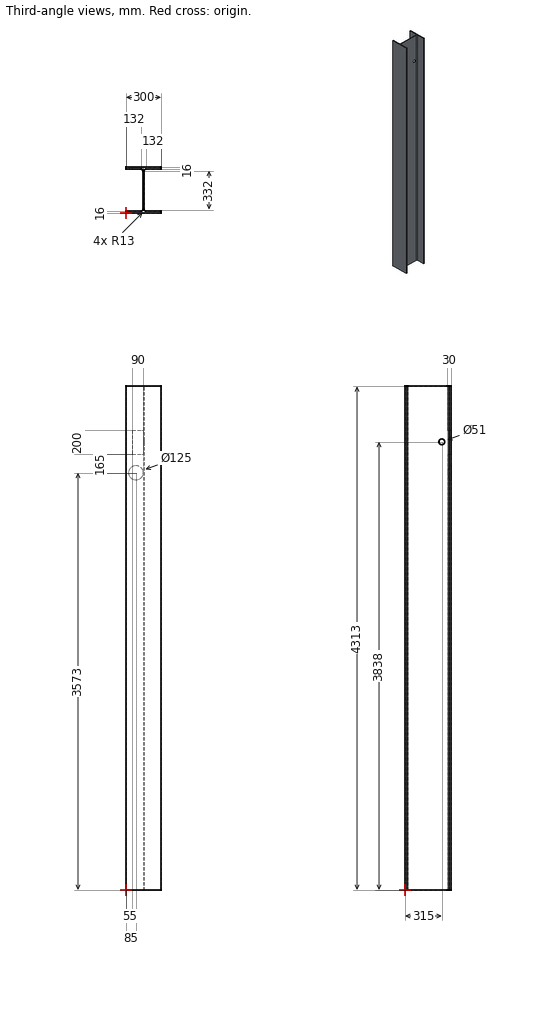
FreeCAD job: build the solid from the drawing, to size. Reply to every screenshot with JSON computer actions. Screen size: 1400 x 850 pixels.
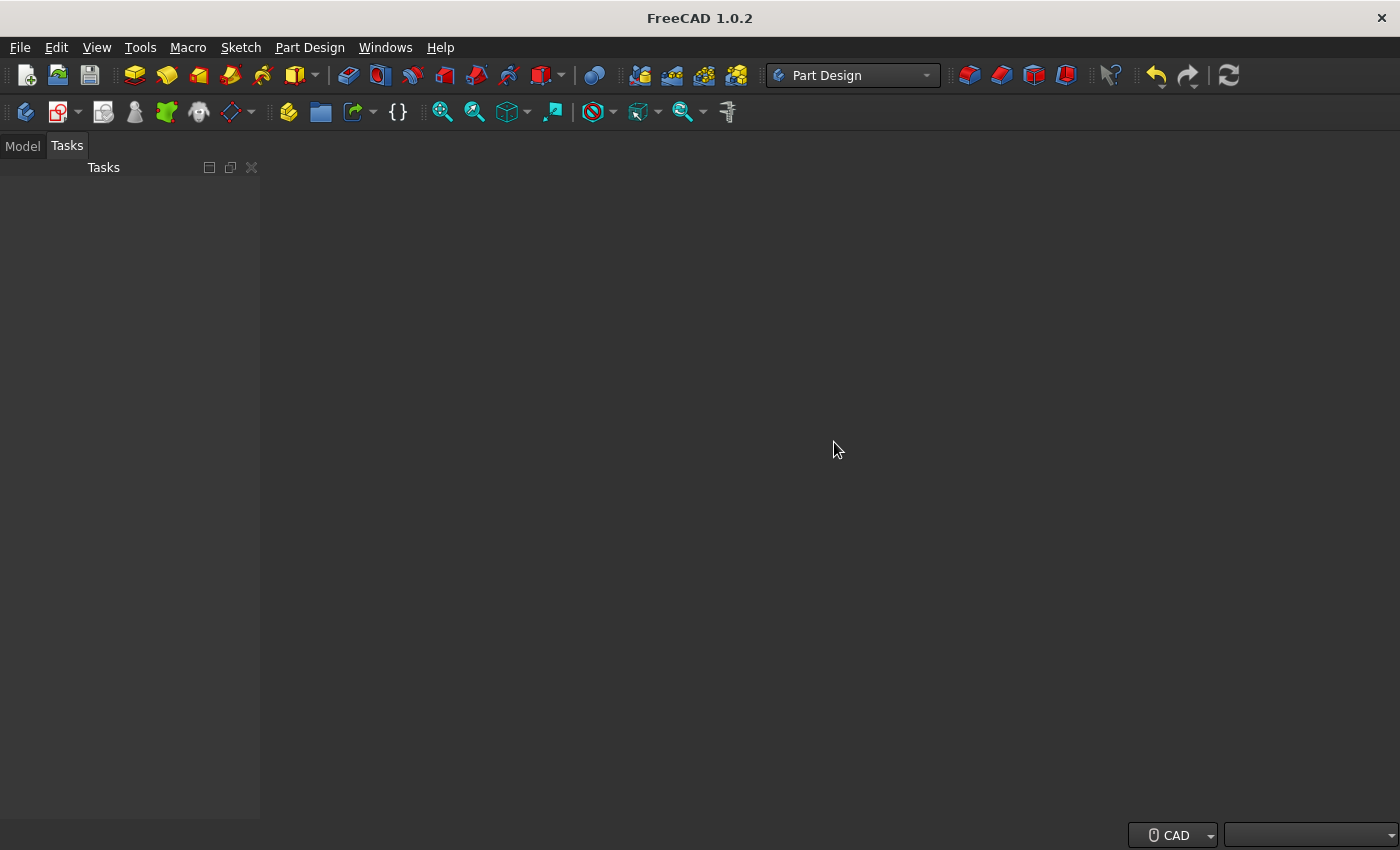
{"action": "left_click", "coordinate": [26, 76]}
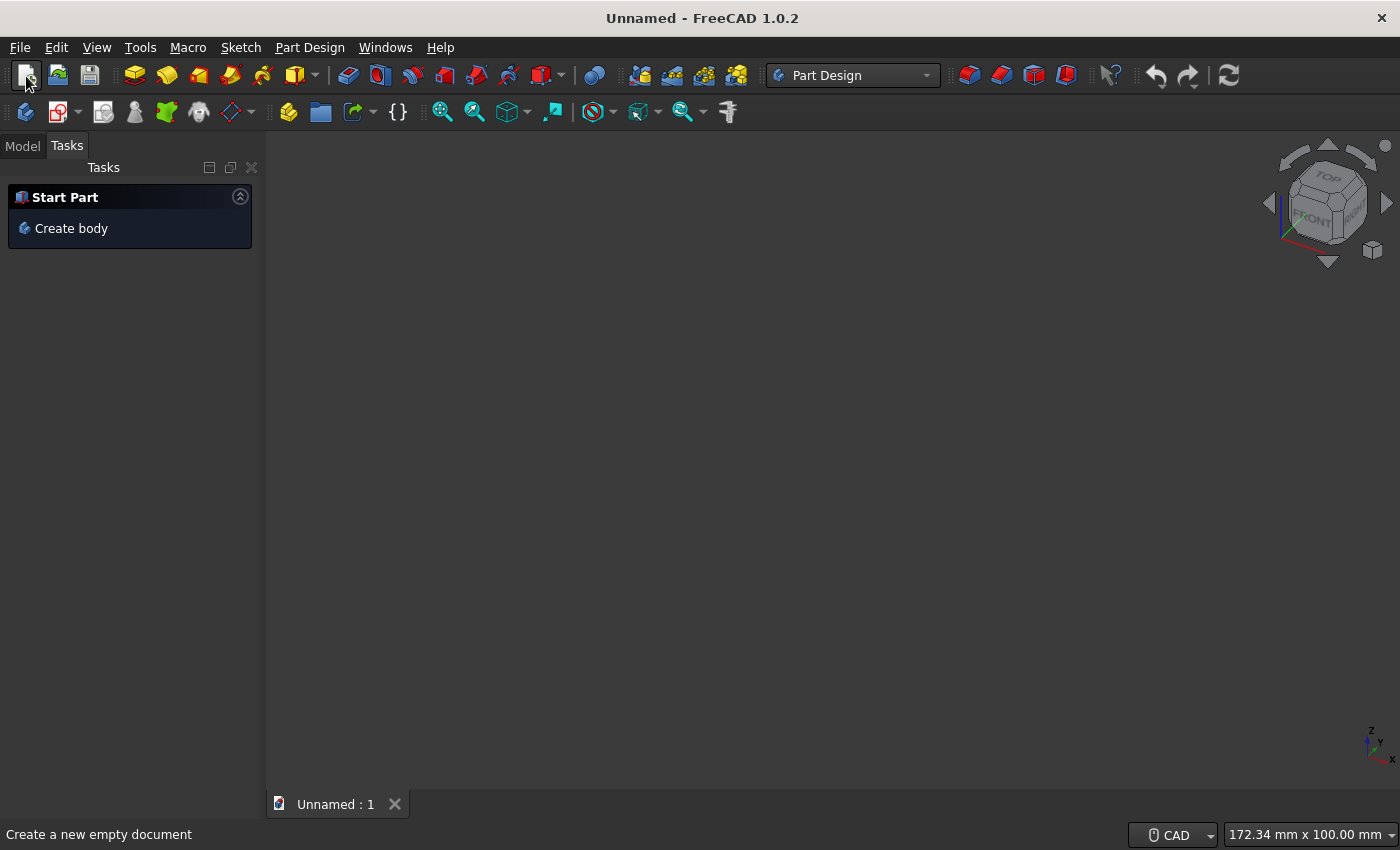
{"action": "left_click", "coordinate": [58, 112]}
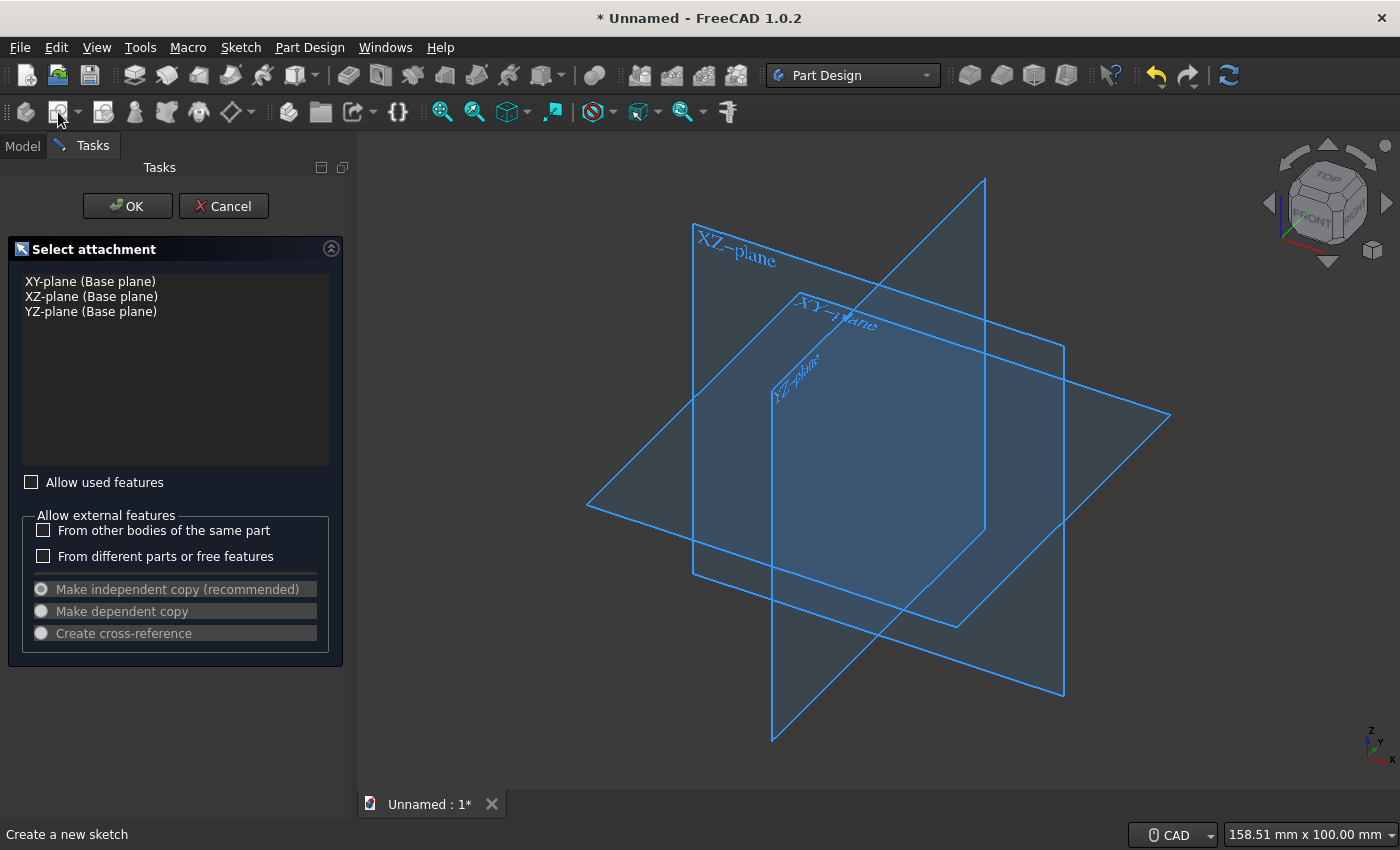
{"action": "left_click", "coordinate": [82, 282]}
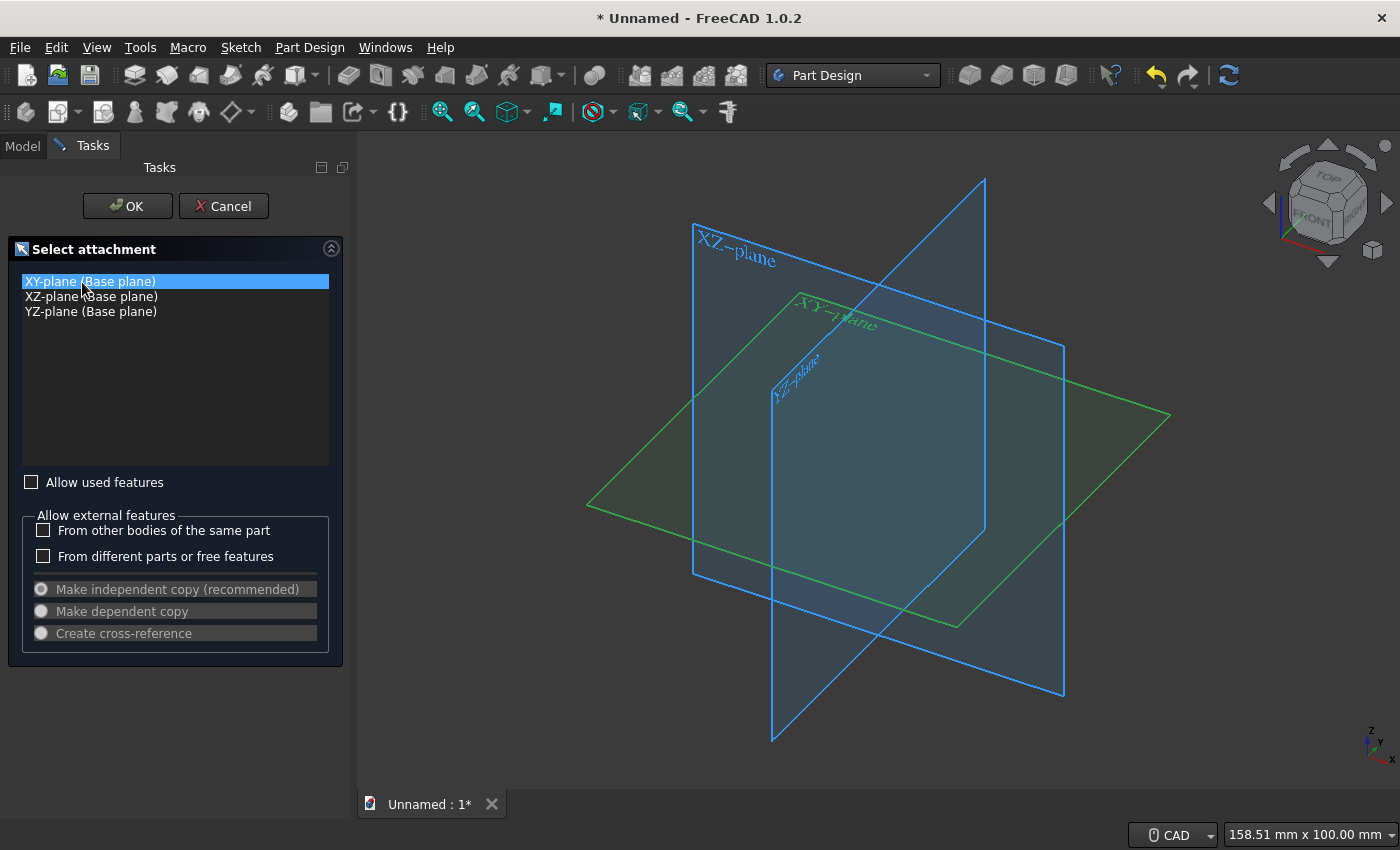
{"action": "left_click", "coordinate": [128, 206]}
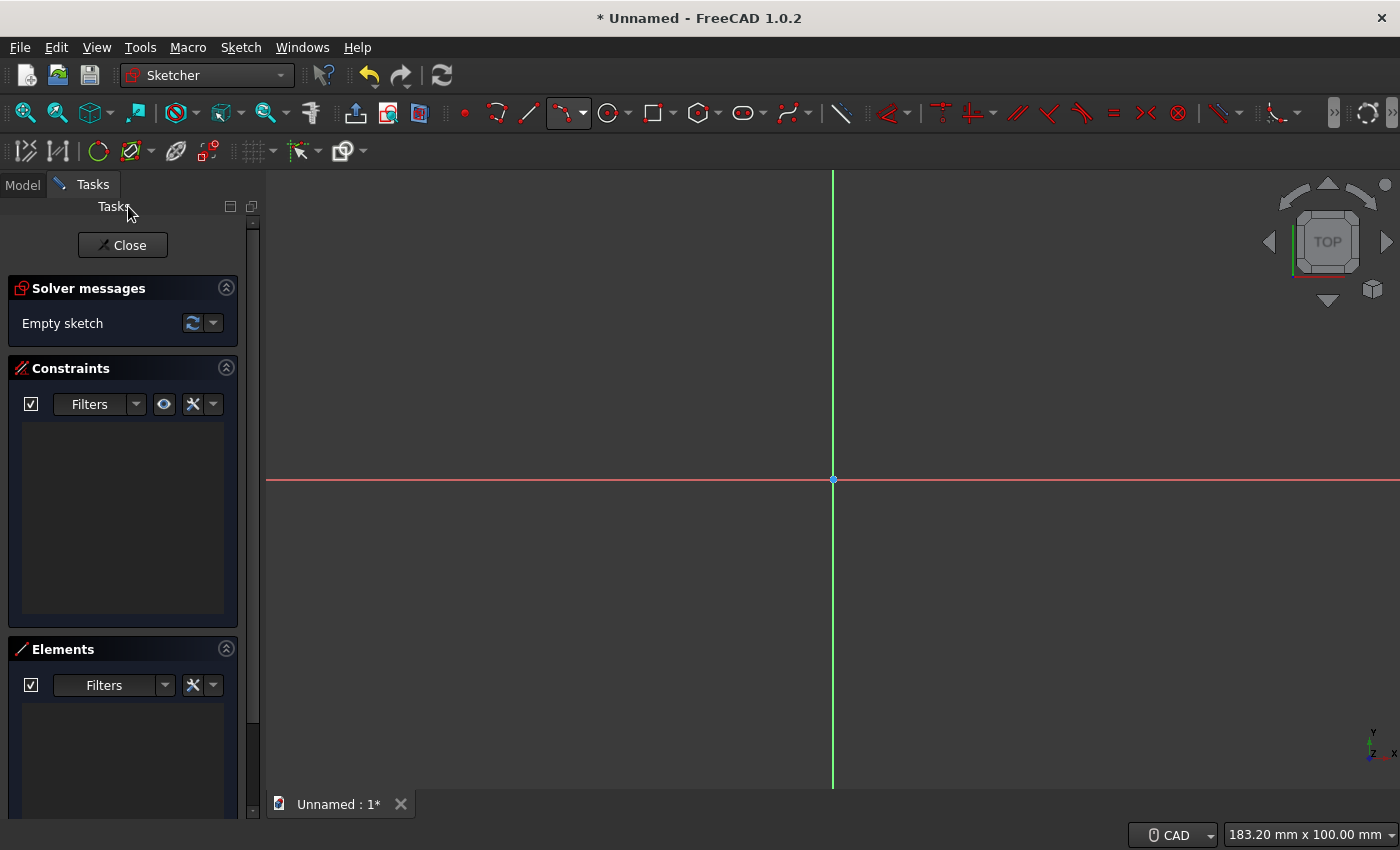
{"action": "scroll", "coordinate": [567, 719], "scroll_direction": "down", "scroll_amount": 9}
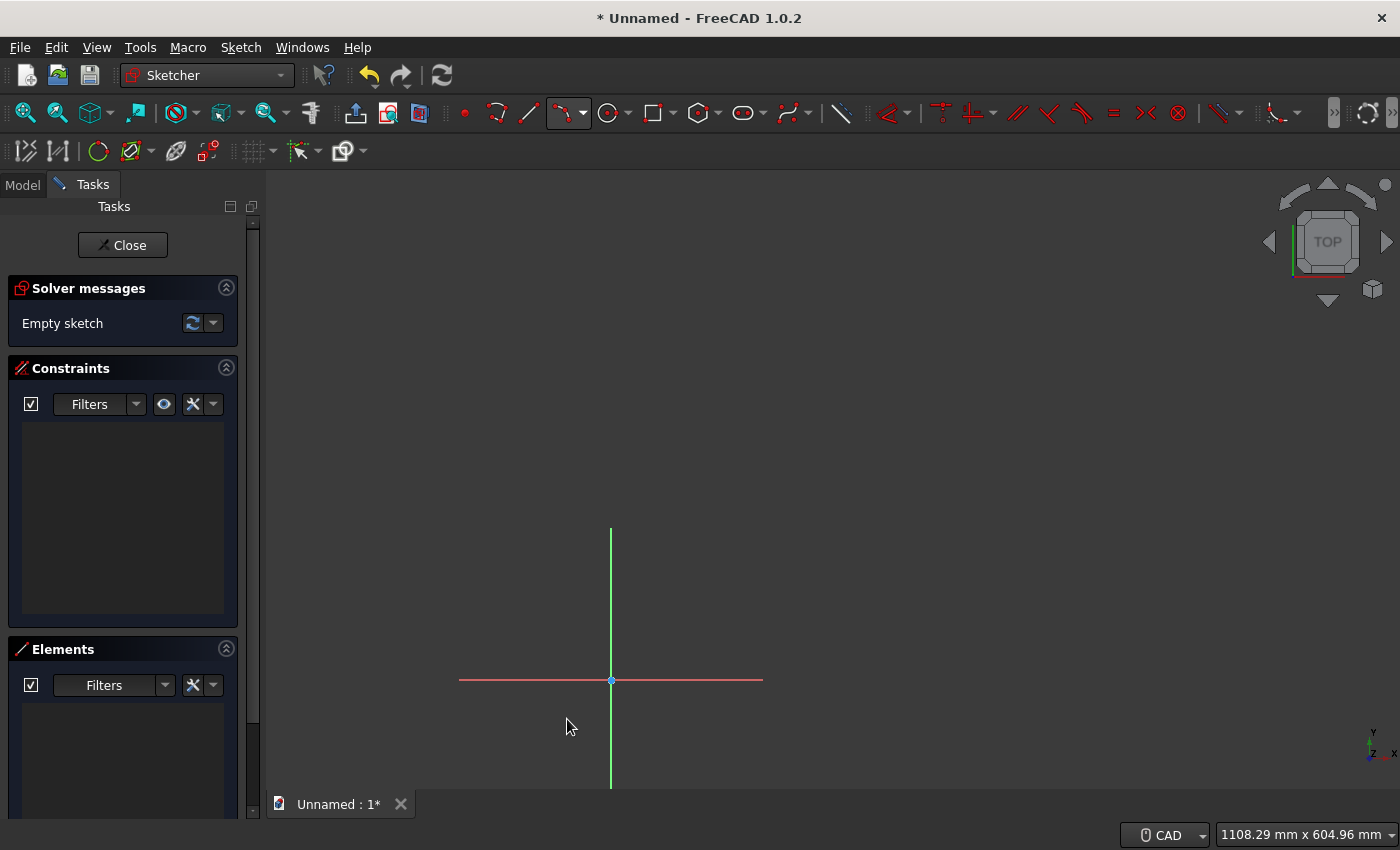
{"action": "key", "text": "g l"}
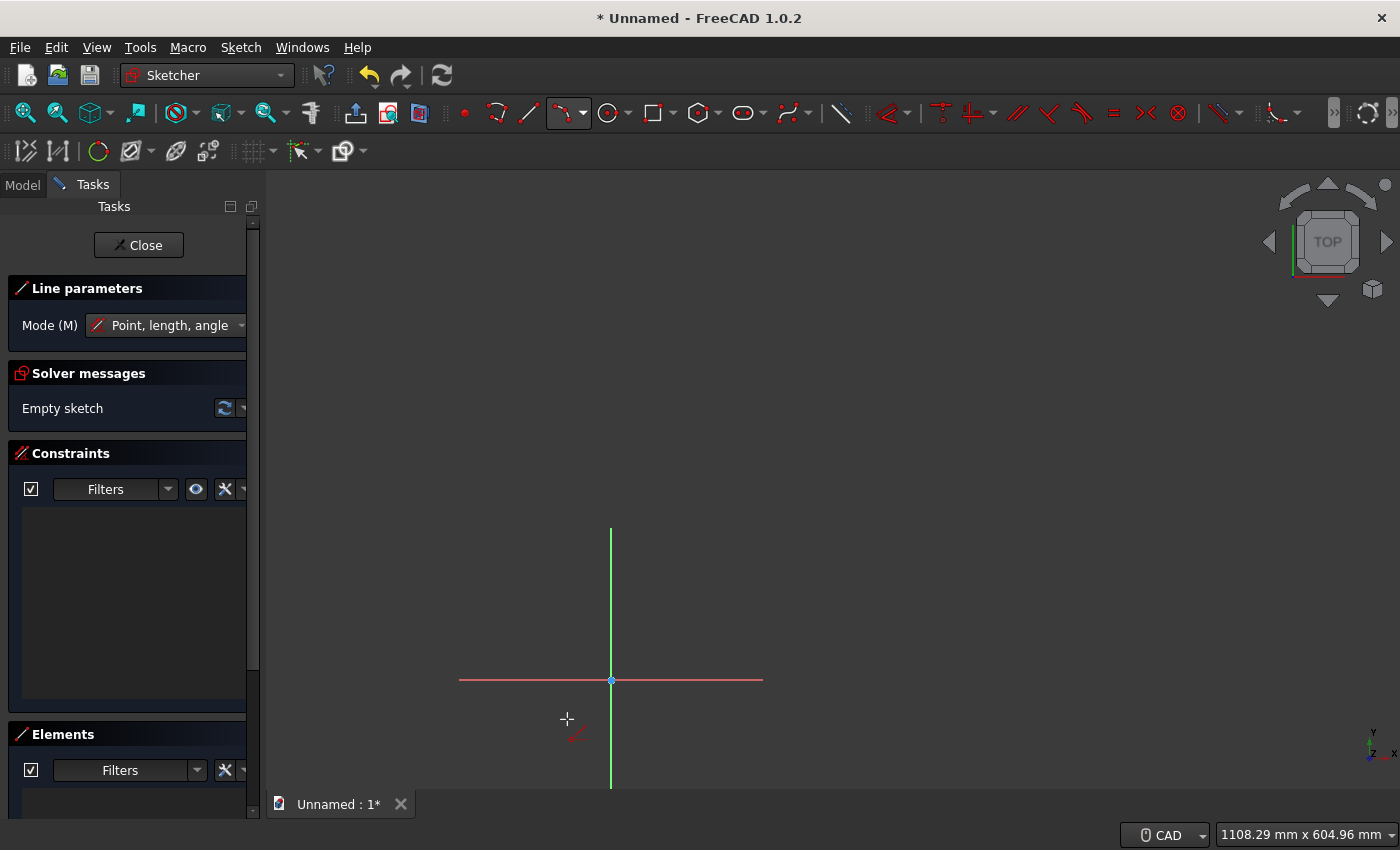
{"action": "left_click", "coordinate": [770, 650]}
{"action": "left_click", "coordinate": [770, 311]}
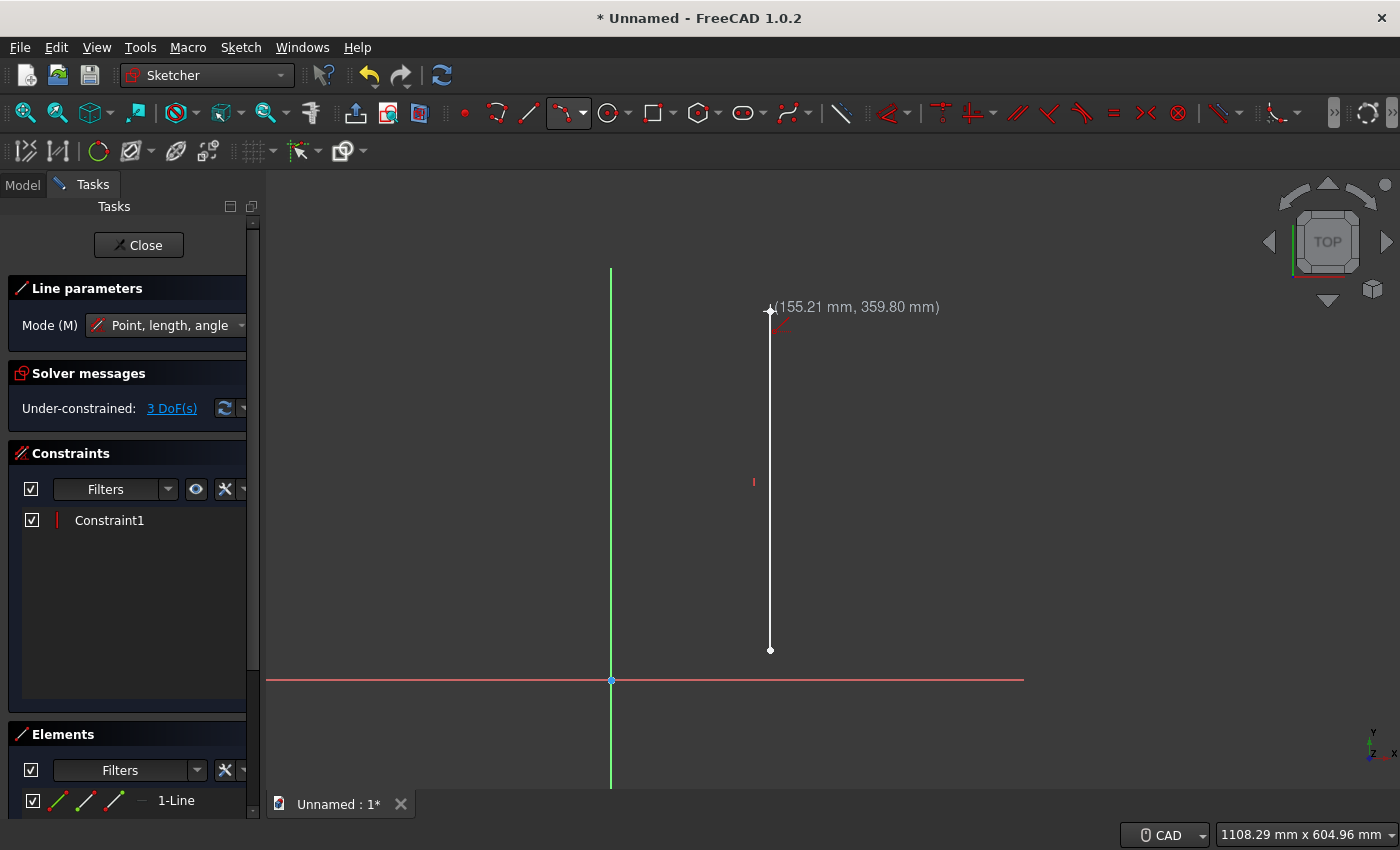
{"action": "left_click", "coordinate": [498, 114]}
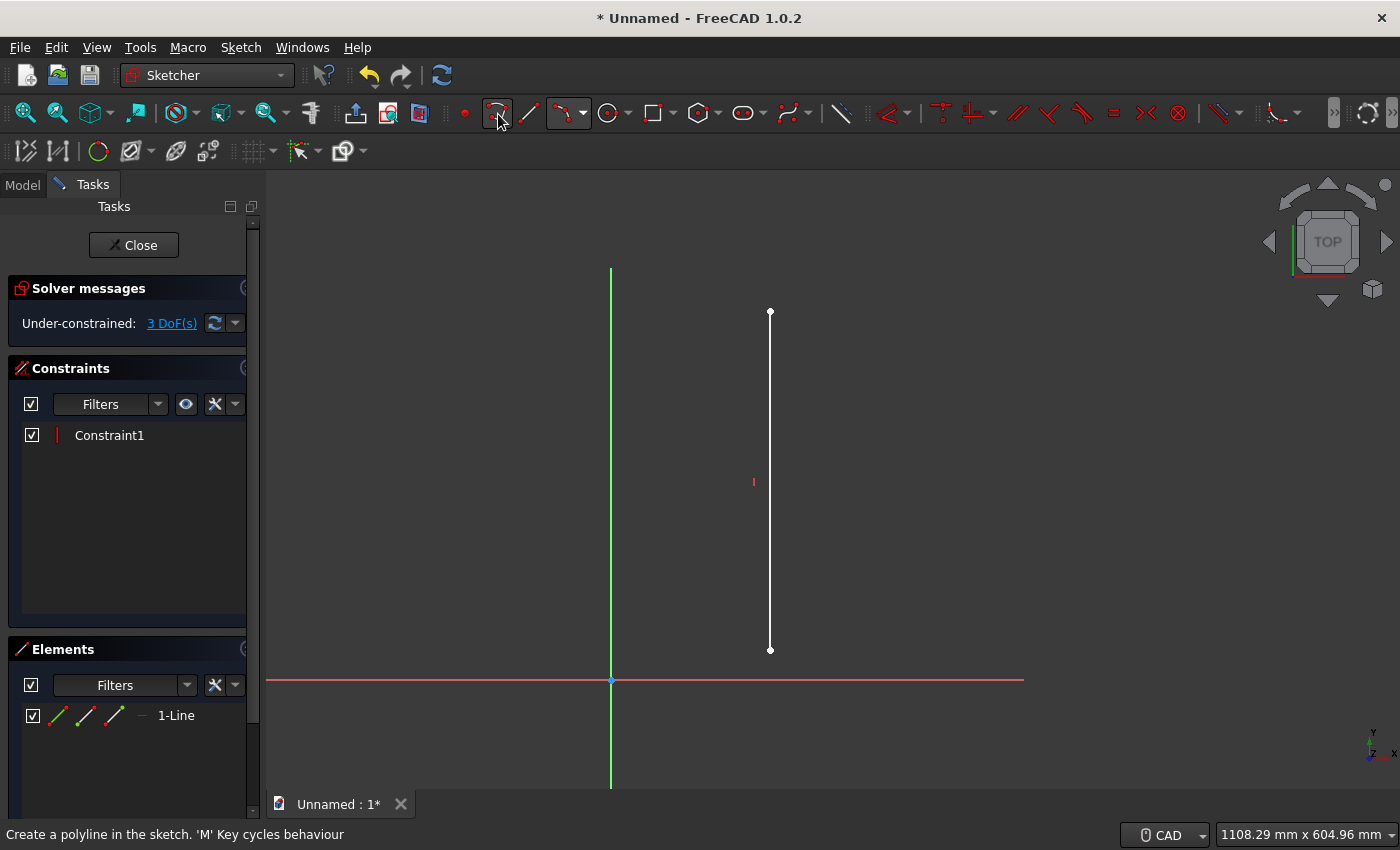
{"action": "left_click", "coordinate": [783, 297]}
{"action": "left_click", "coordinate": [918, 297]}
{"action": "left_click", "coordinate": [918, 281]}
{"action": "left_click", "coordinate": [611, 281]}
{"action": "left_click", "coordinate": [620, 297]}
{"action": "left_click", "coordinate": [746, 297]}
{"action": "right_click", "coordinate": [746, 297]}